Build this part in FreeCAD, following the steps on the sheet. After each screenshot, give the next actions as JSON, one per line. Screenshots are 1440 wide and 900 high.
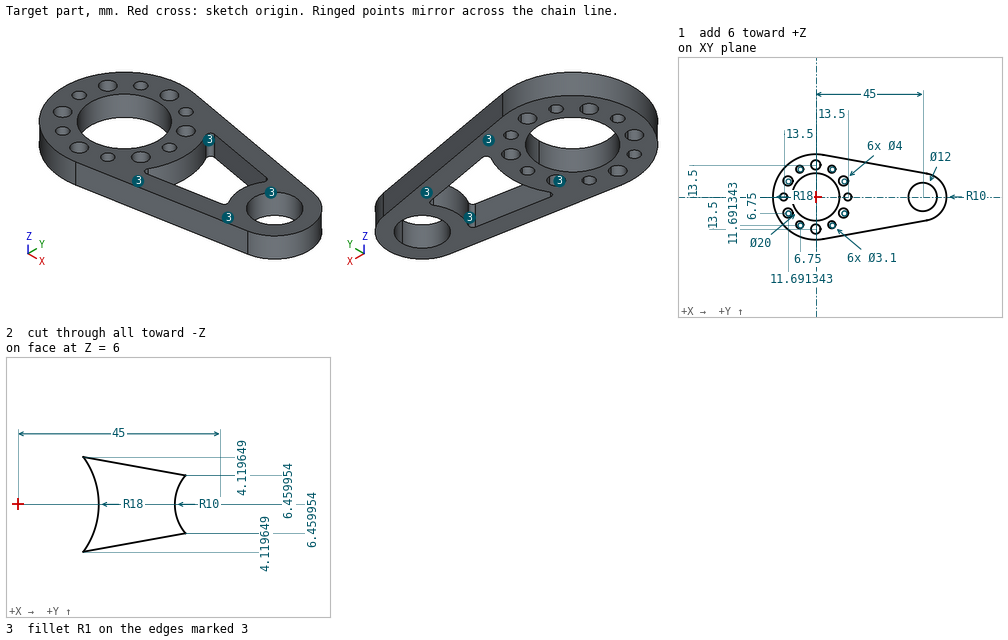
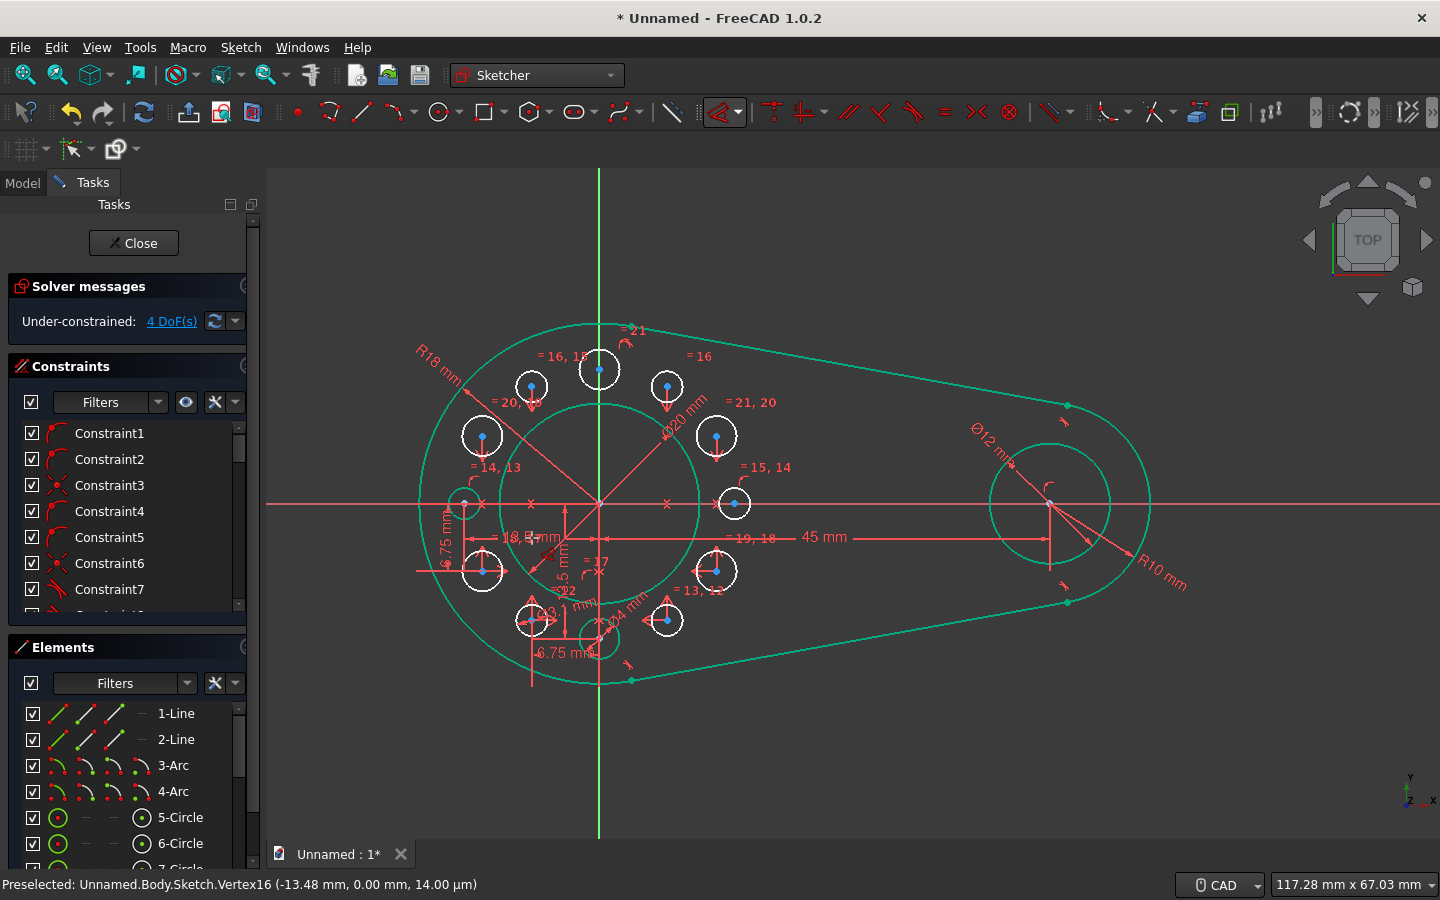
{"action": "left_click", "coordinate": [735, 504]}
{"action": "left_click", "coordinate": [667, 538]}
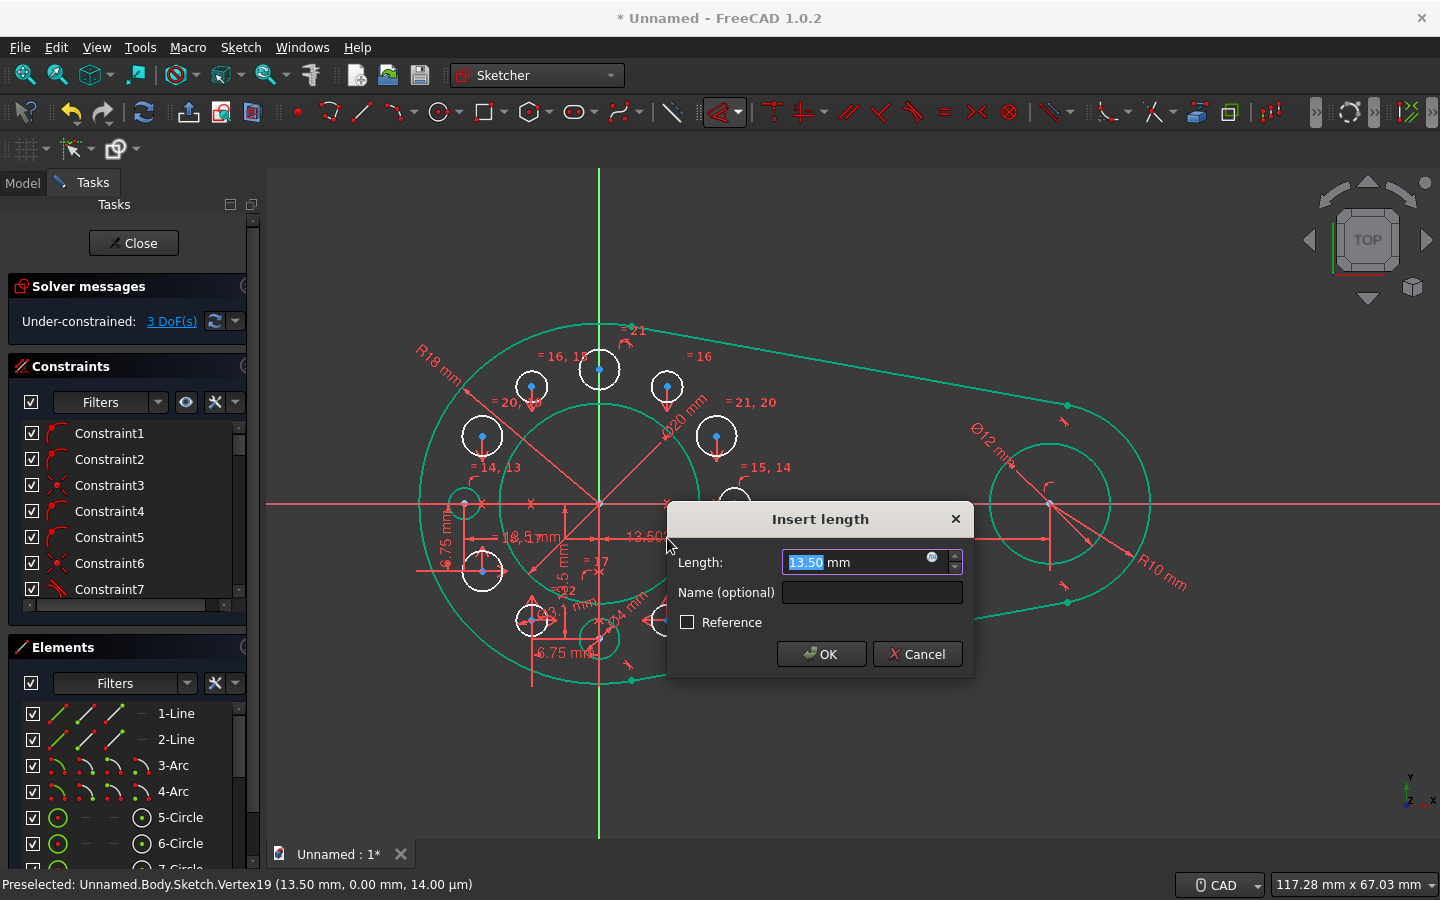
{"action": "type", "text": "13.5"}
{"action": "key", "text": "Return"}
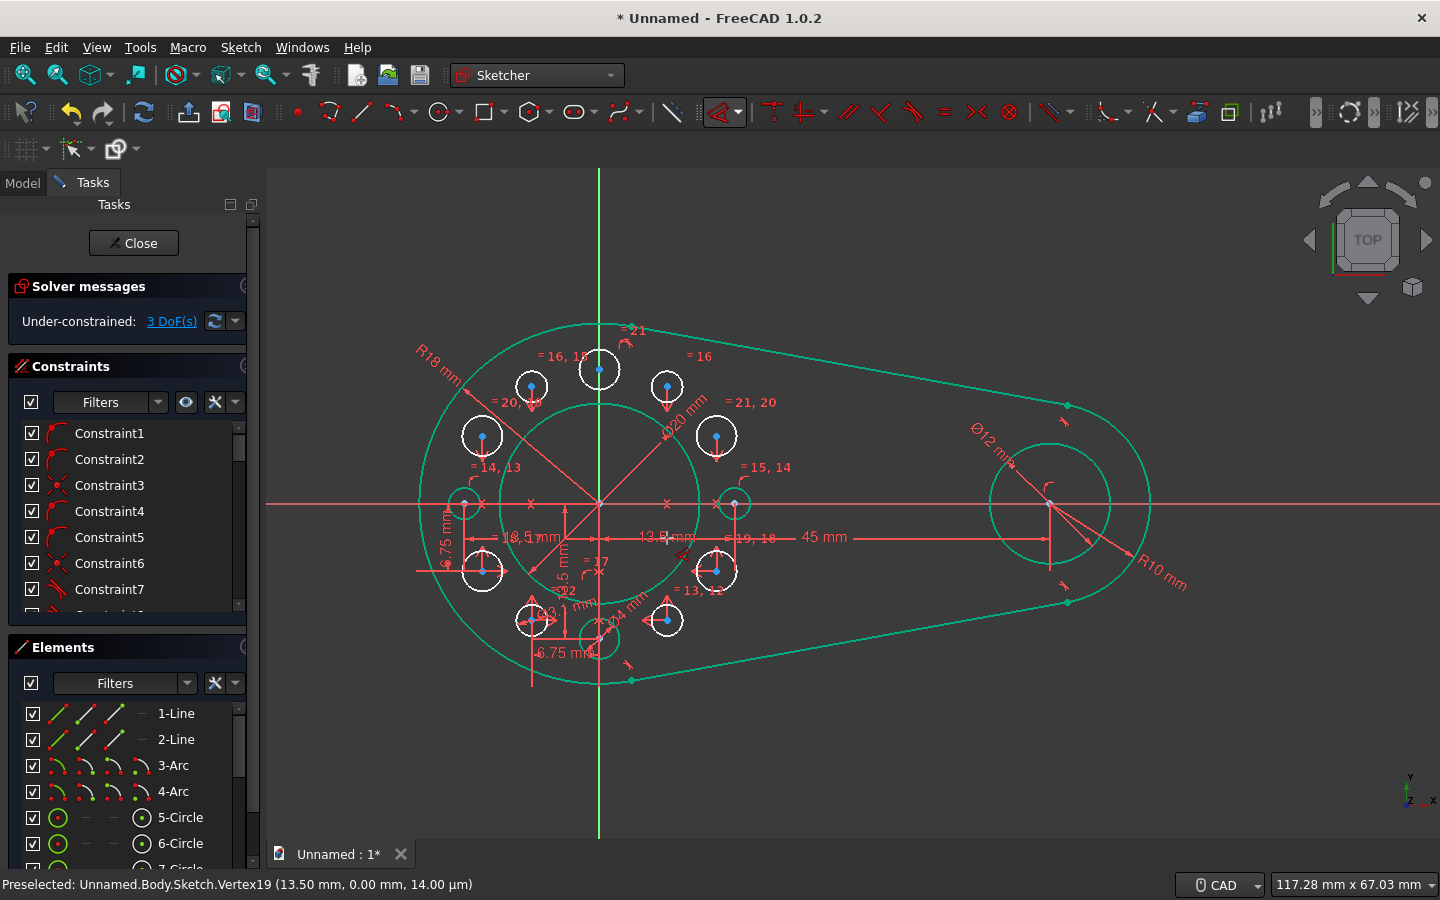
{"action": "left_click", "coordinate": [599, 370]}
{"action": "left_click", "coordinate": [565, 437]}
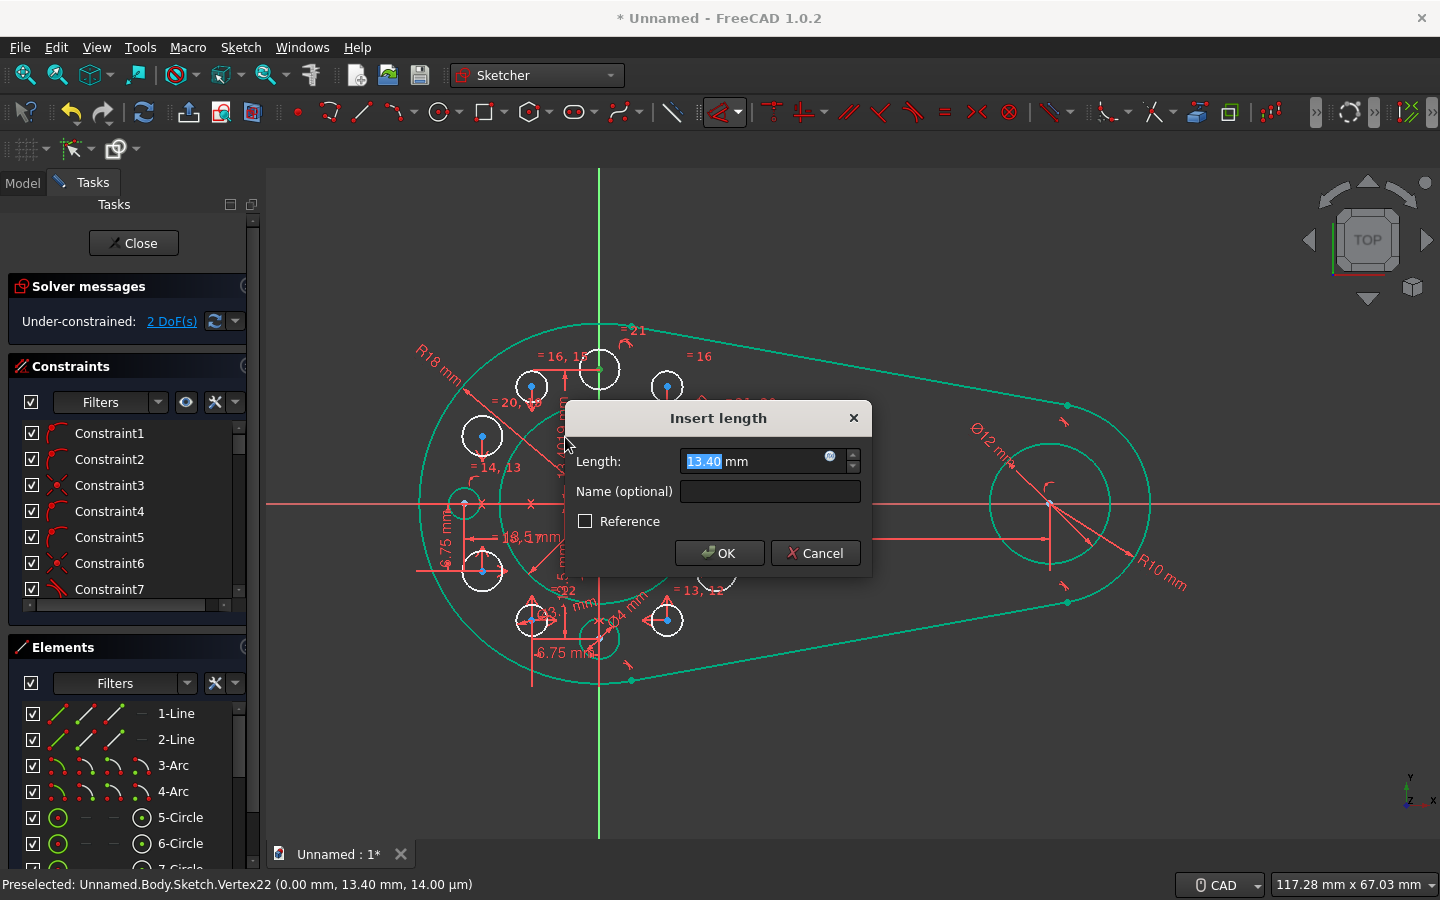
{"action": "type", "text": "13.5"}
{"action": "key", "text": "Return"}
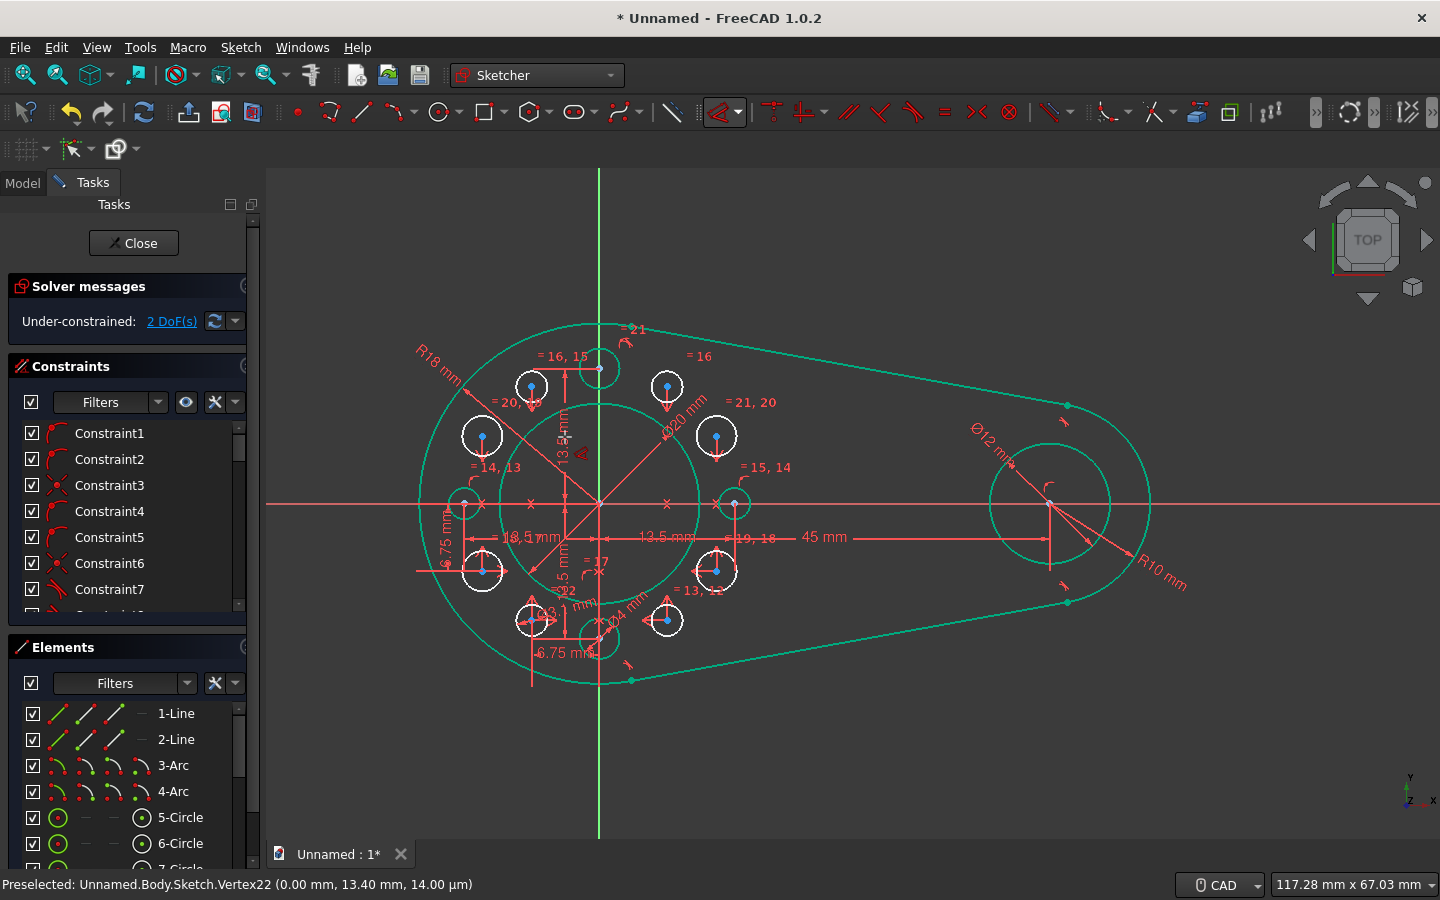
{"action": "left_click", "coordinate": [532, 620]}
{"action": "left_click", "coordinate": [657, 562]}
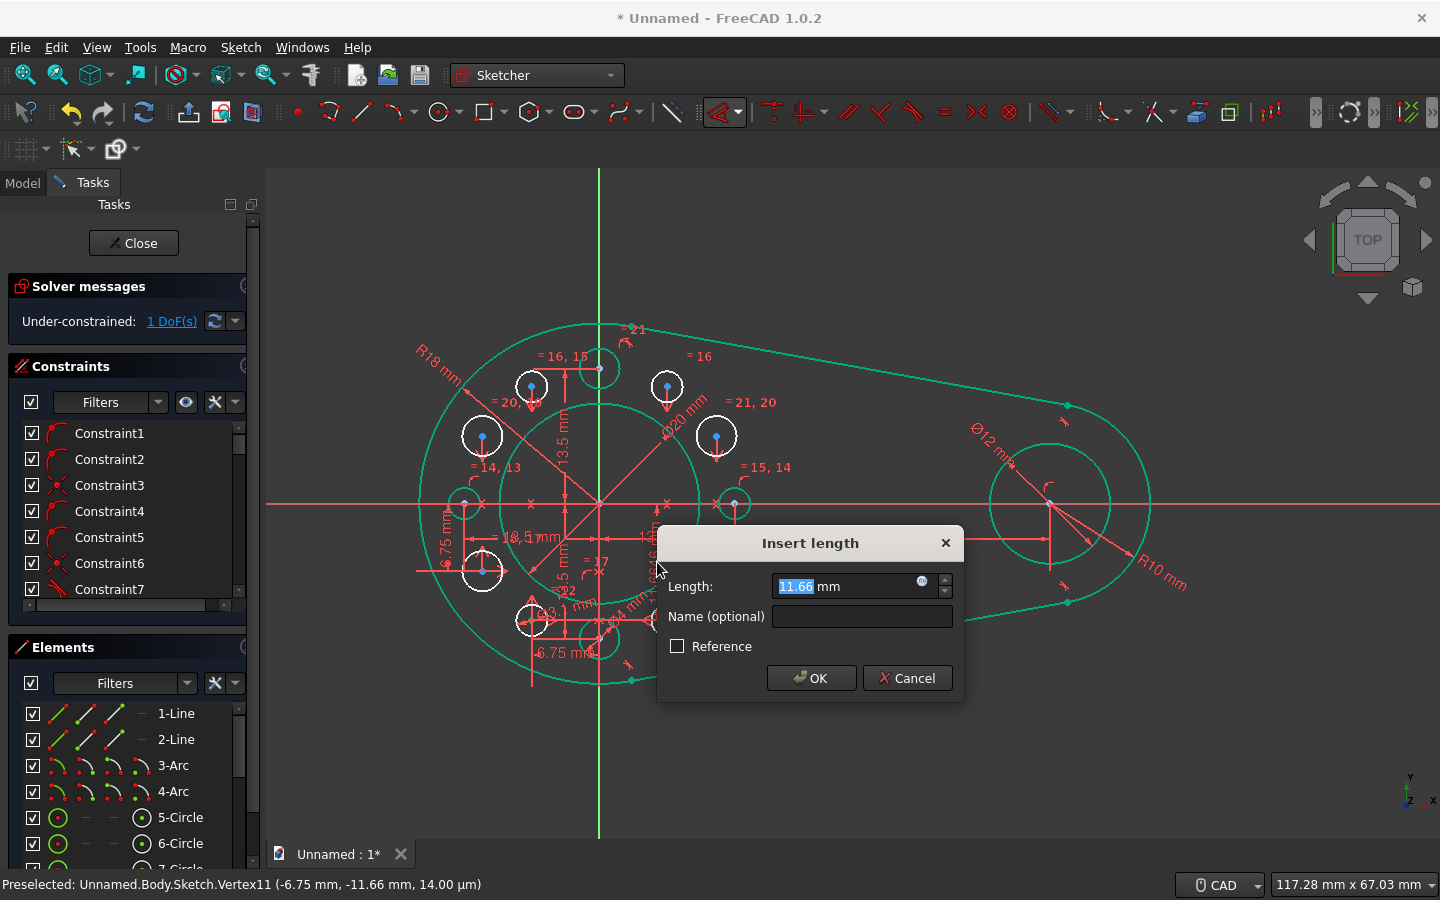
{"action": "type", "text": "11.691343"}
{"action": "key", "text": "Return"}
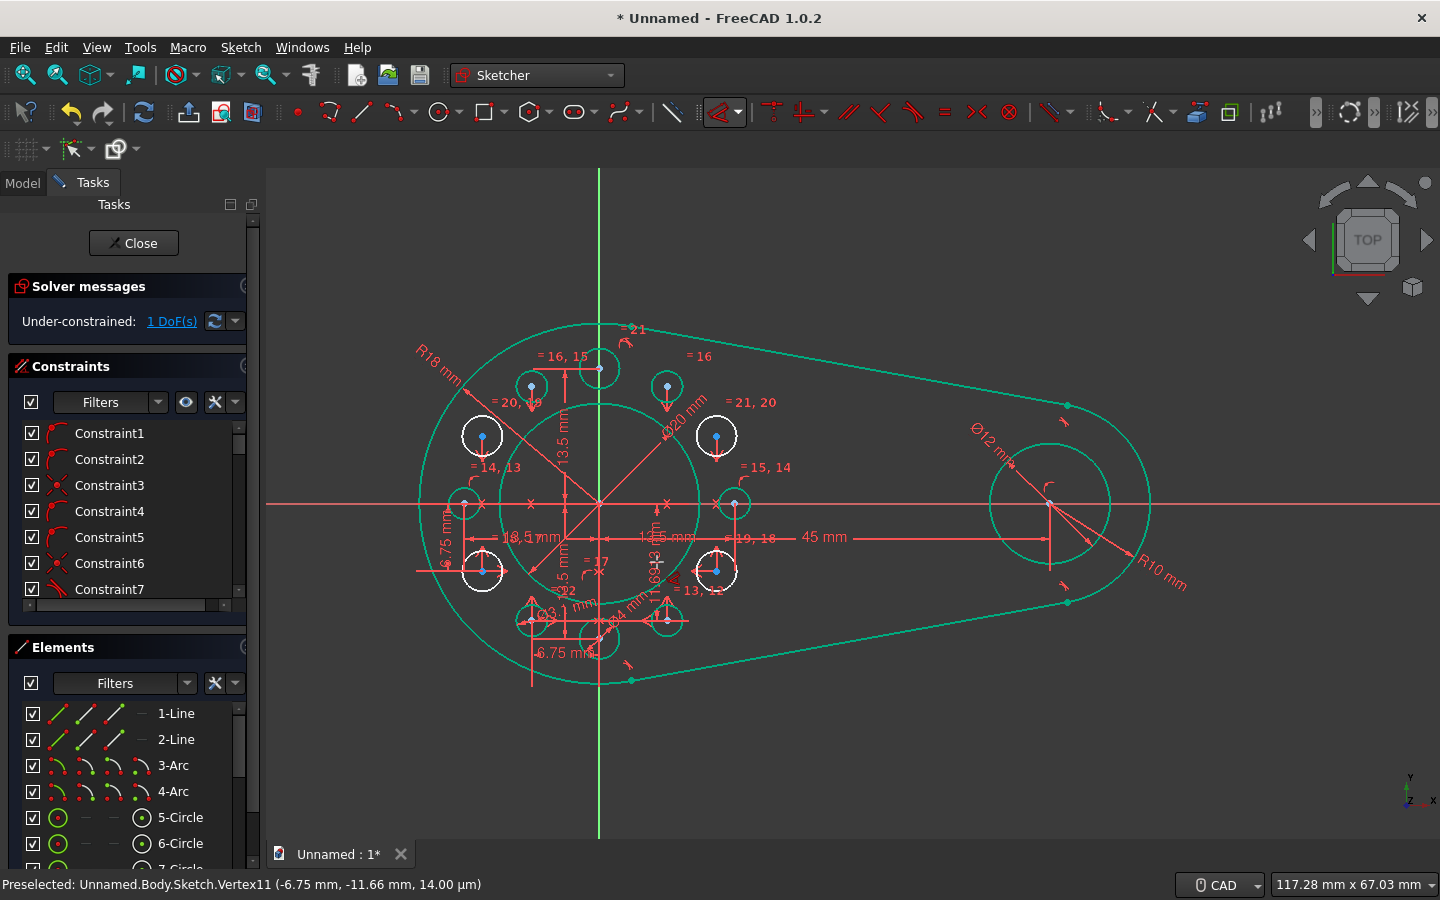
{"action": "left_click", "coordinate": [482, 571]}
{"action": "left_click", "coordinate": [541, 470]}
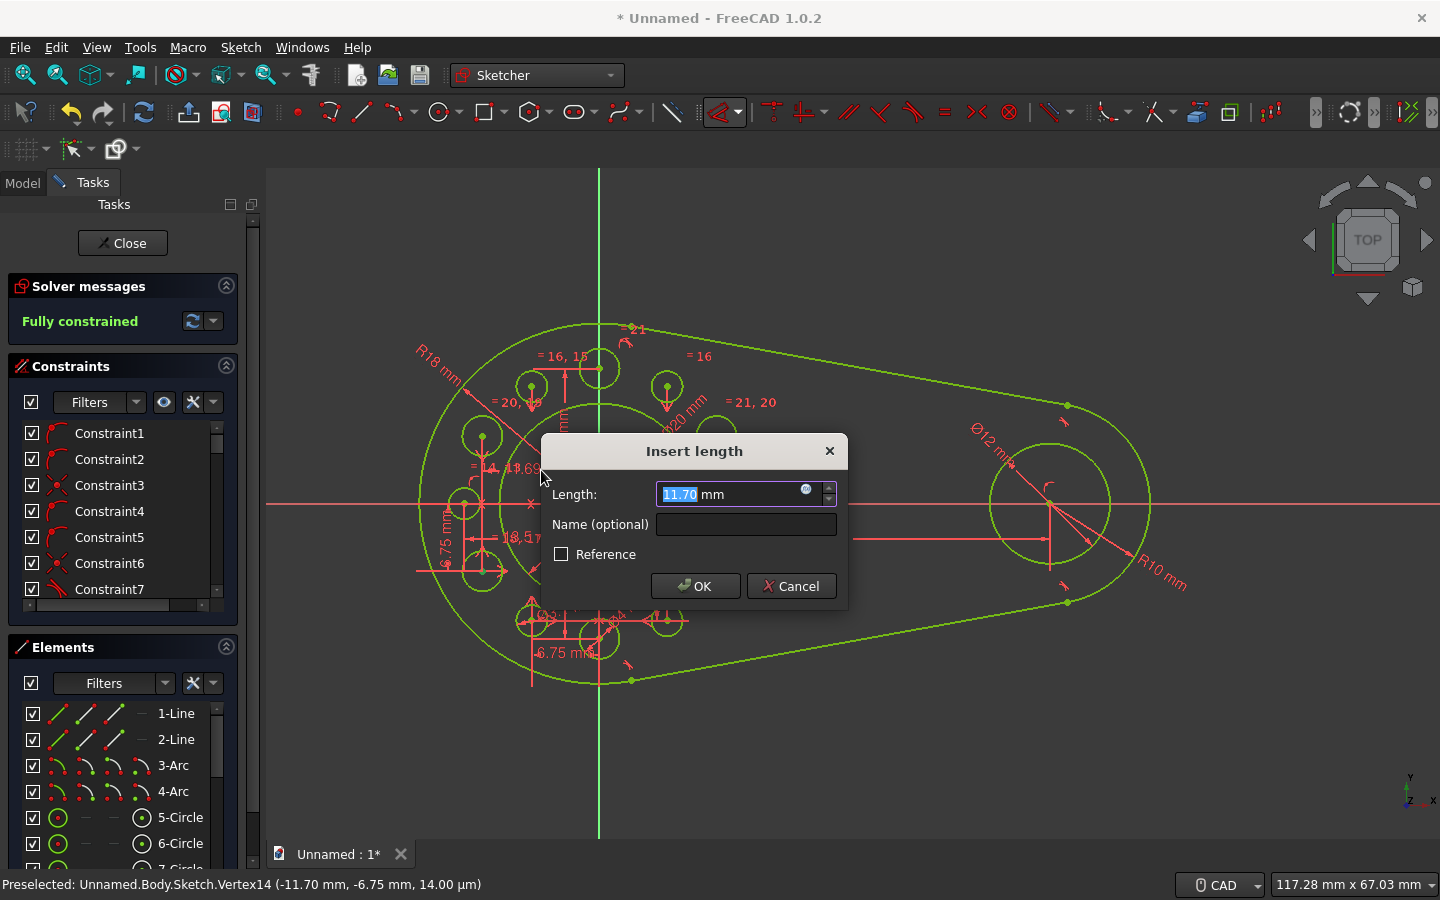
{"action": "type", "text": "11.691343"}
{"action": "key", "text": "Return"}
{"action": "key", "text": "Escape"}